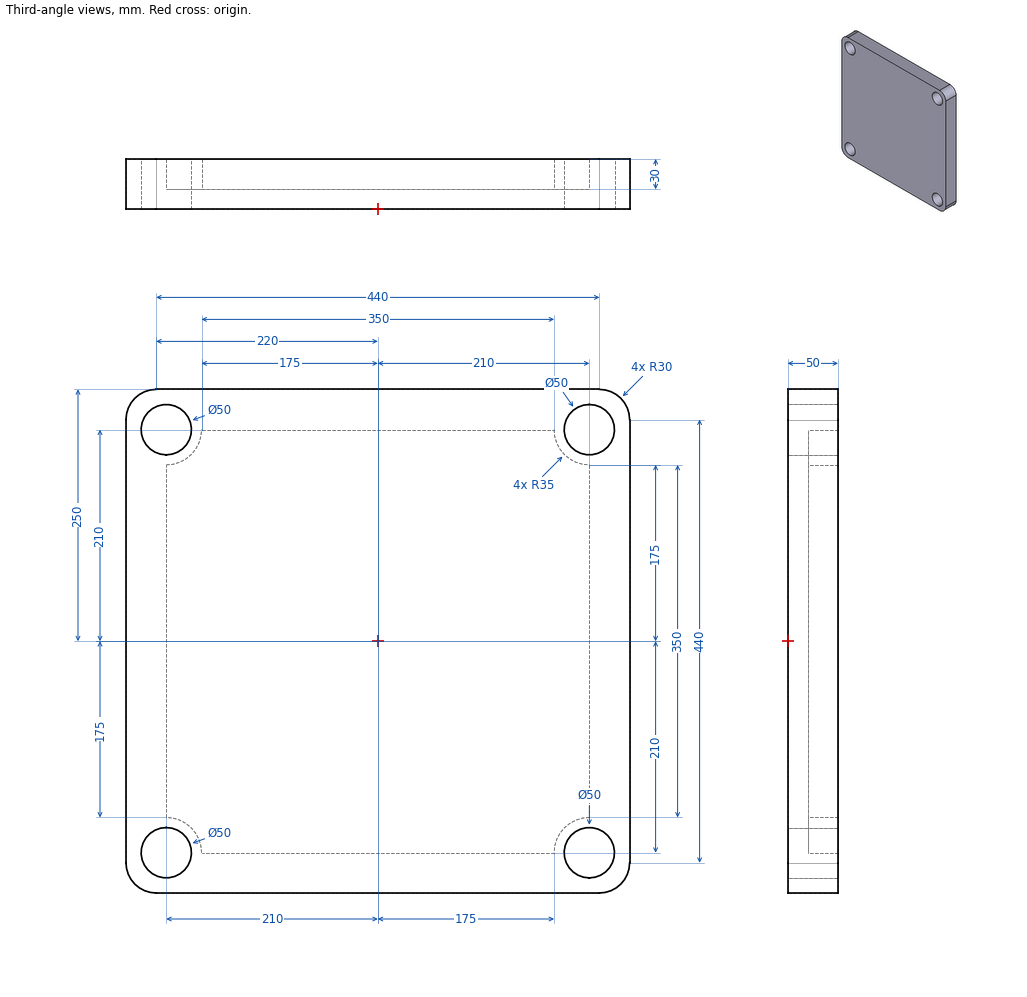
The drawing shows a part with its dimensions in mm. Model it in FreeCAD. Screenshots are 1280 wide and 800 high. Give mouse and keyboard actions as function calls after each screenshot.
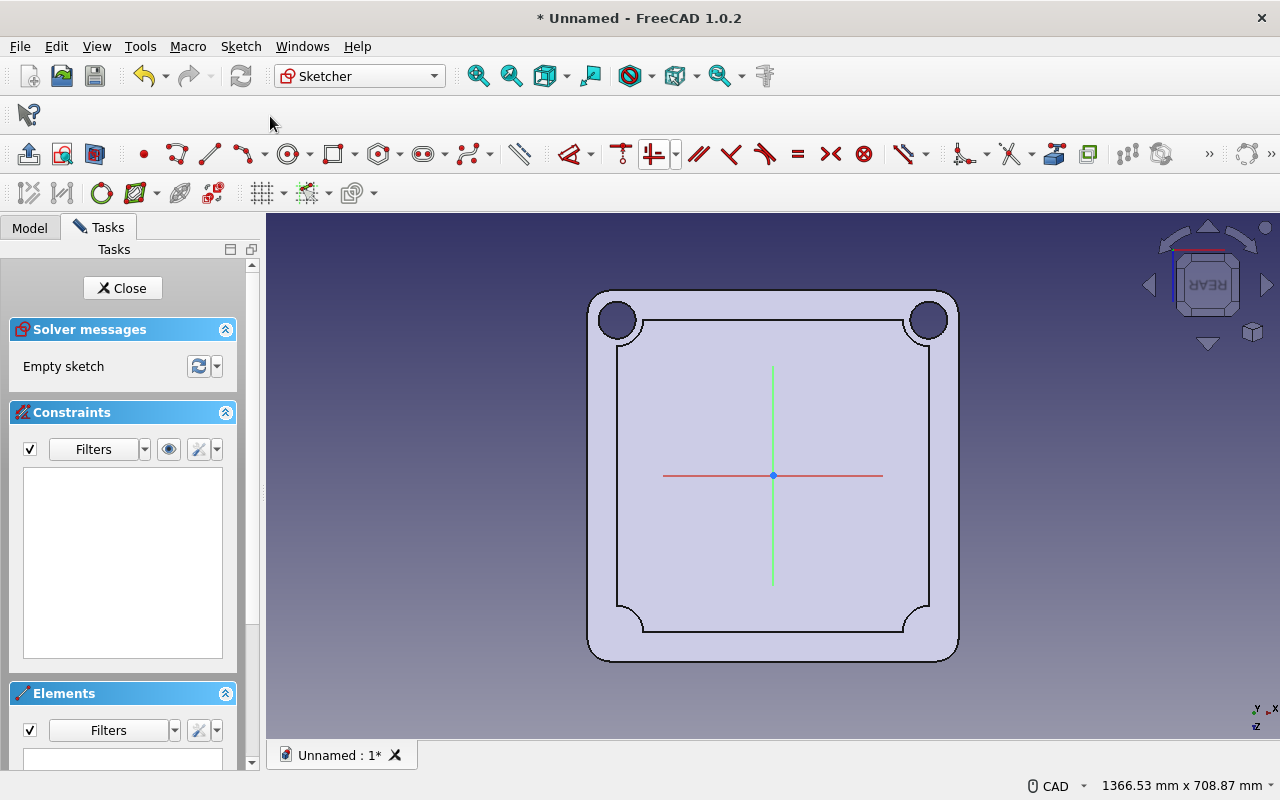
scroll(957, 651, up, 11)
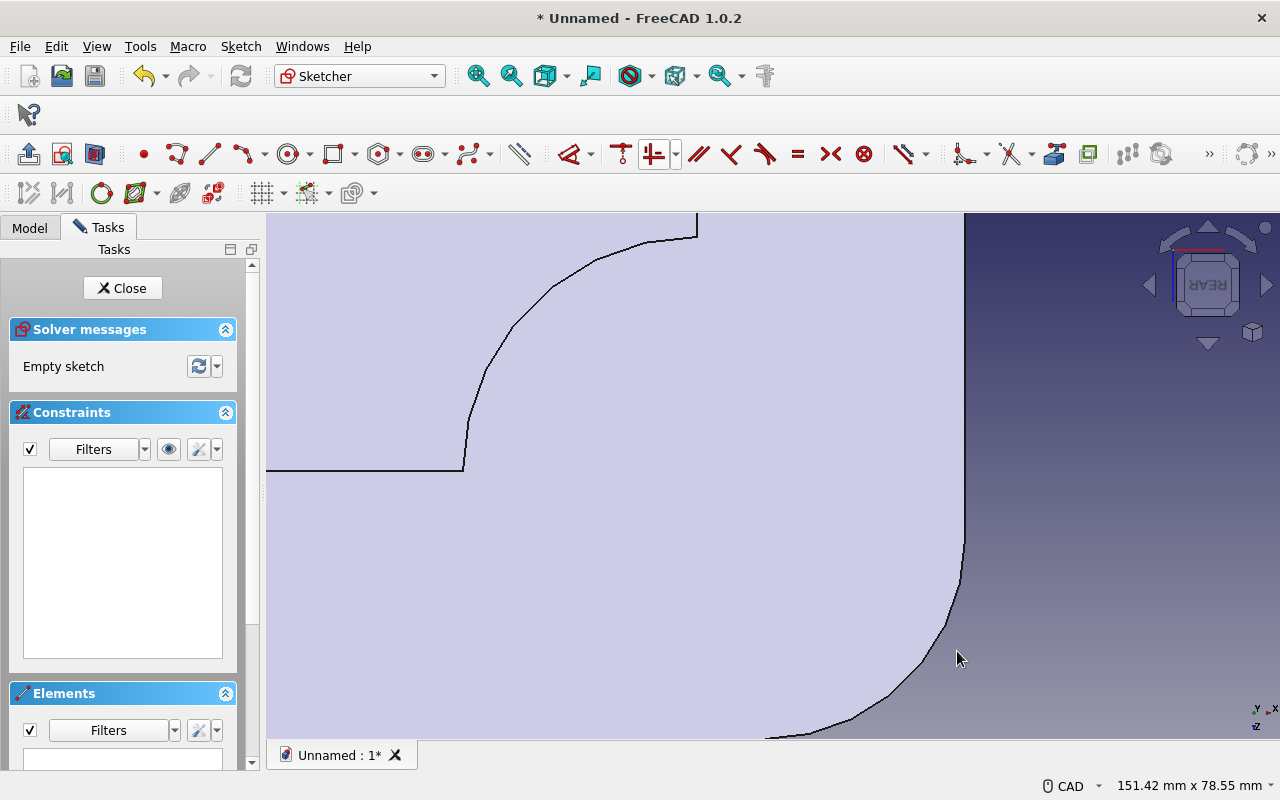
click(288, 154)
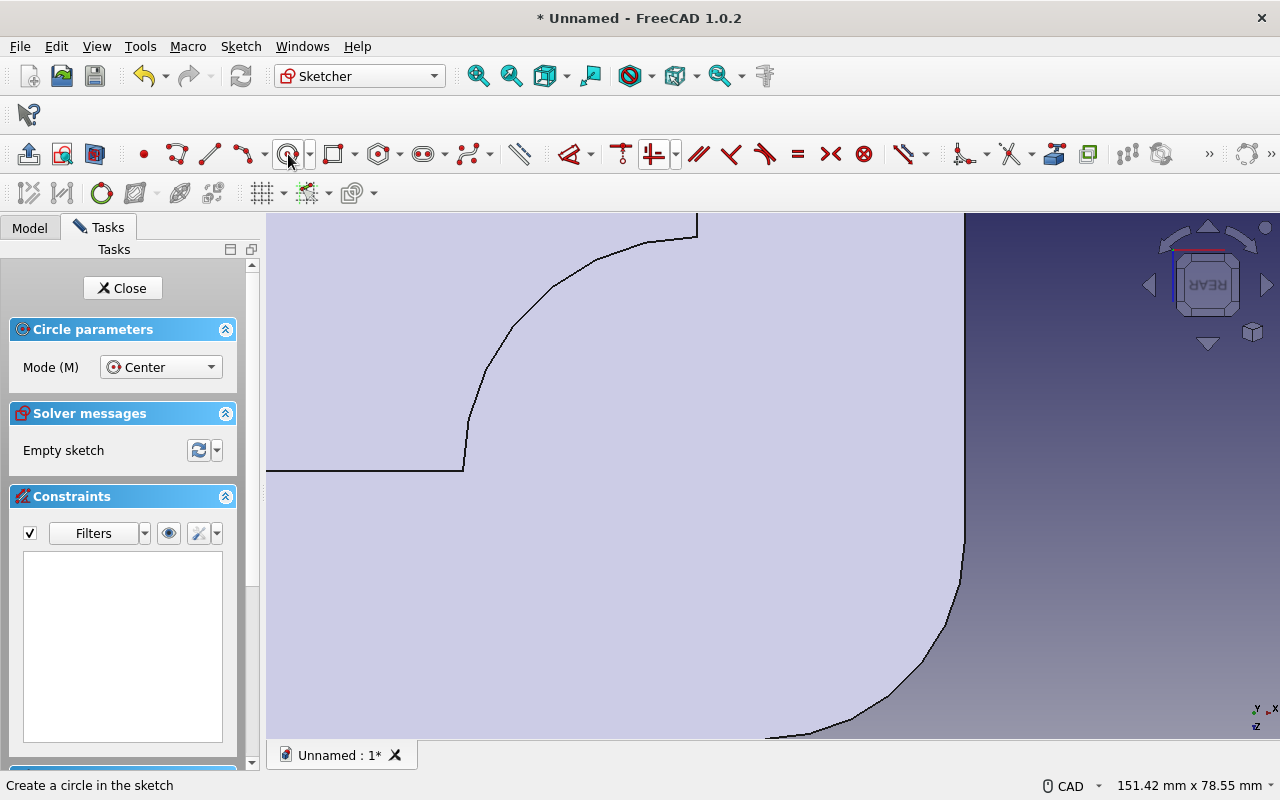
click(697, 471)
move(816, 353)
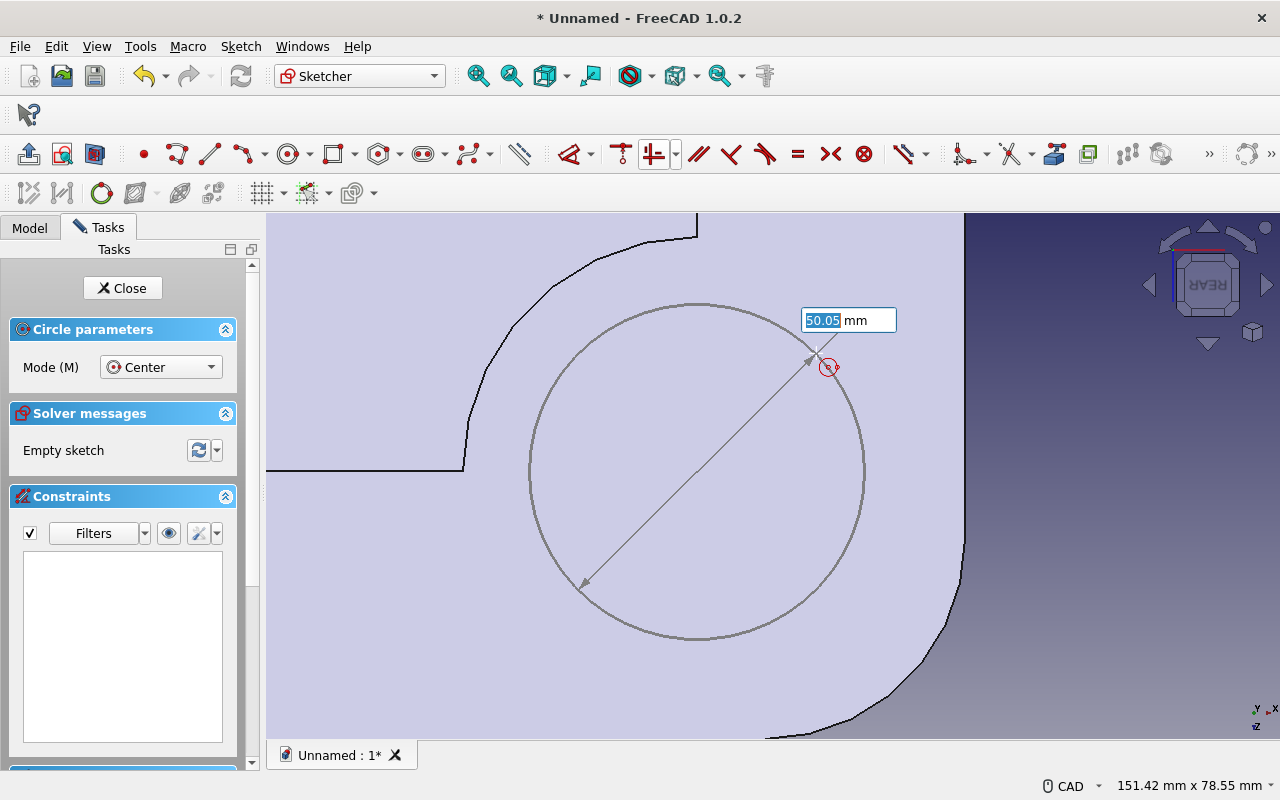
text(50)
key(Return)
key(Escape)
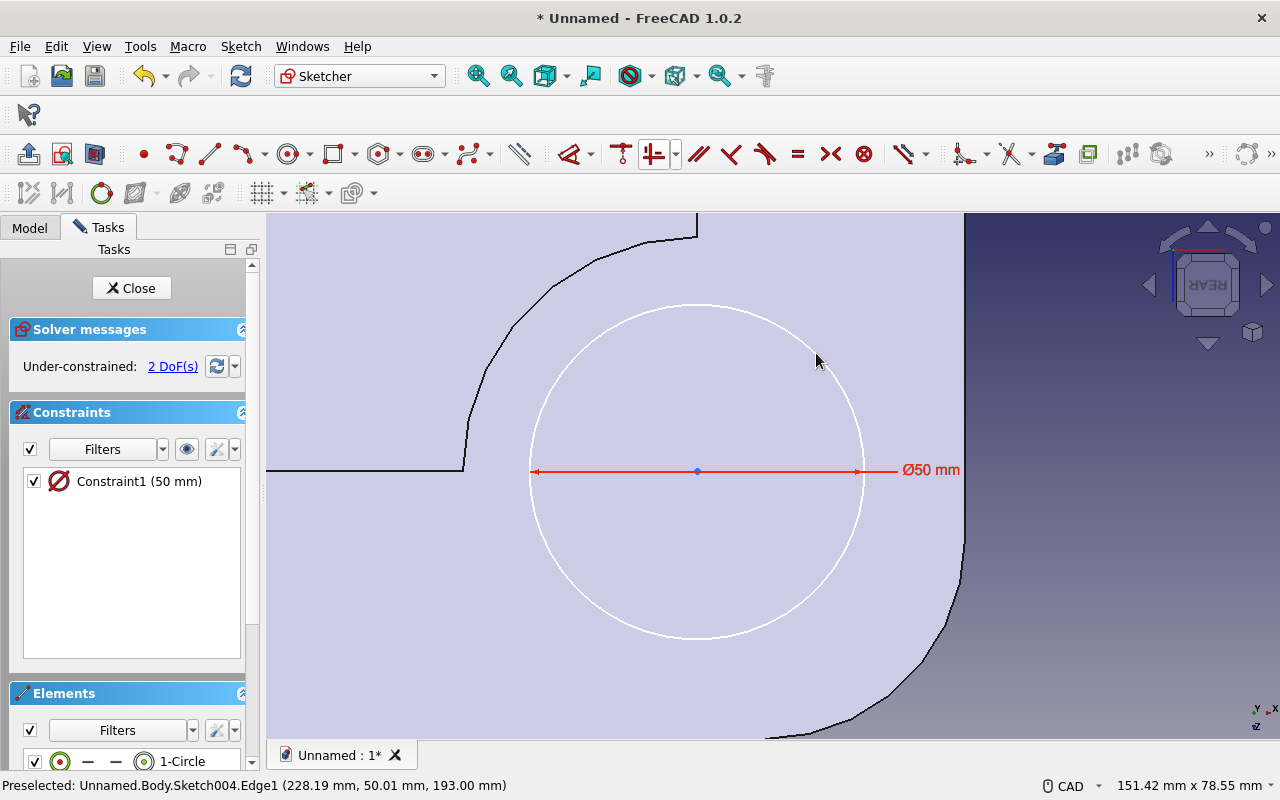
click(568, 154)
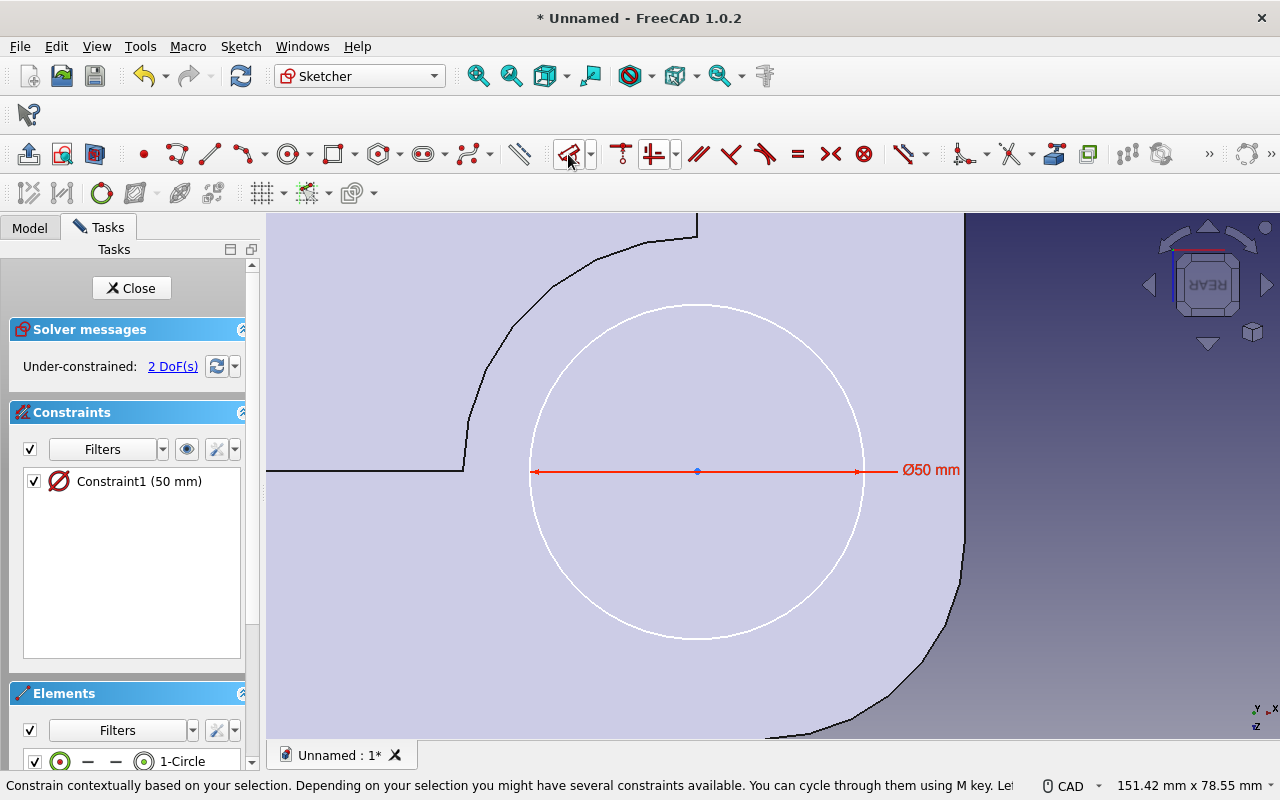
click(697, 472)
click(495, 506)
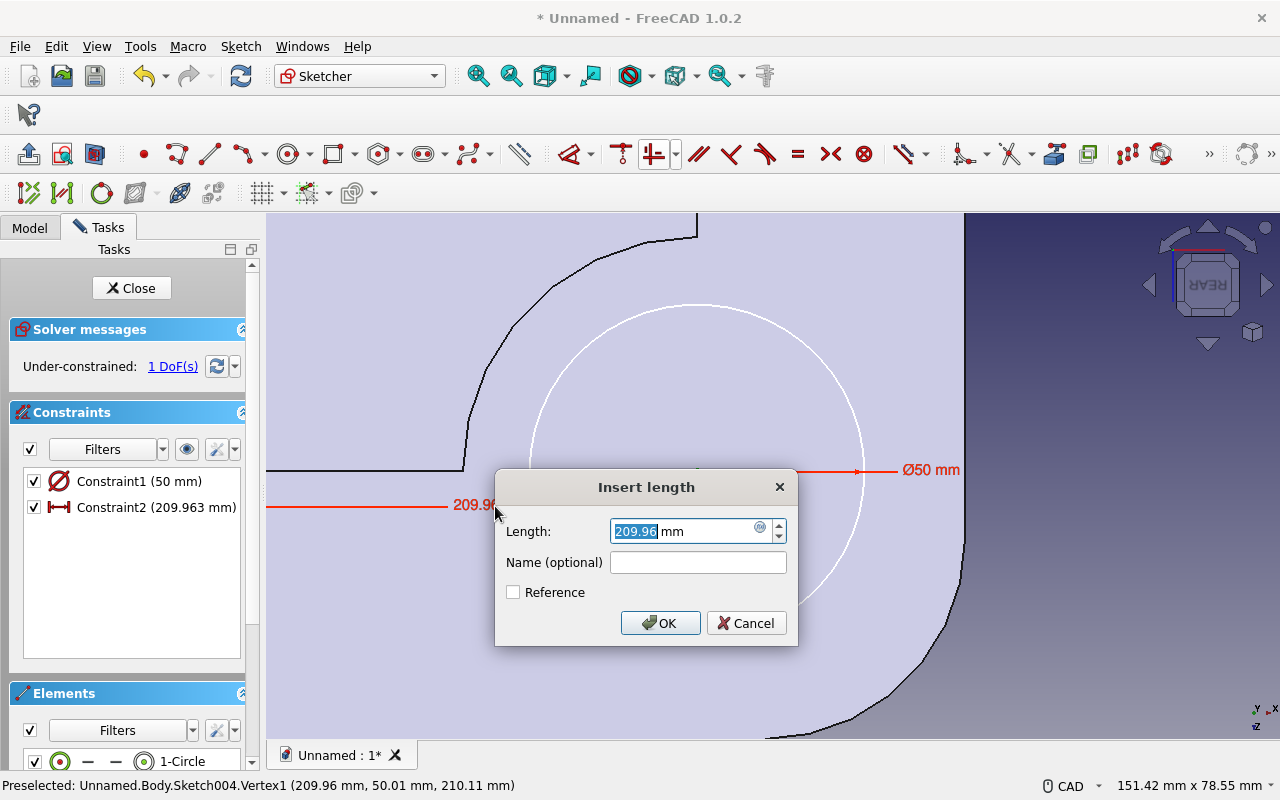
text(210)
key(Return)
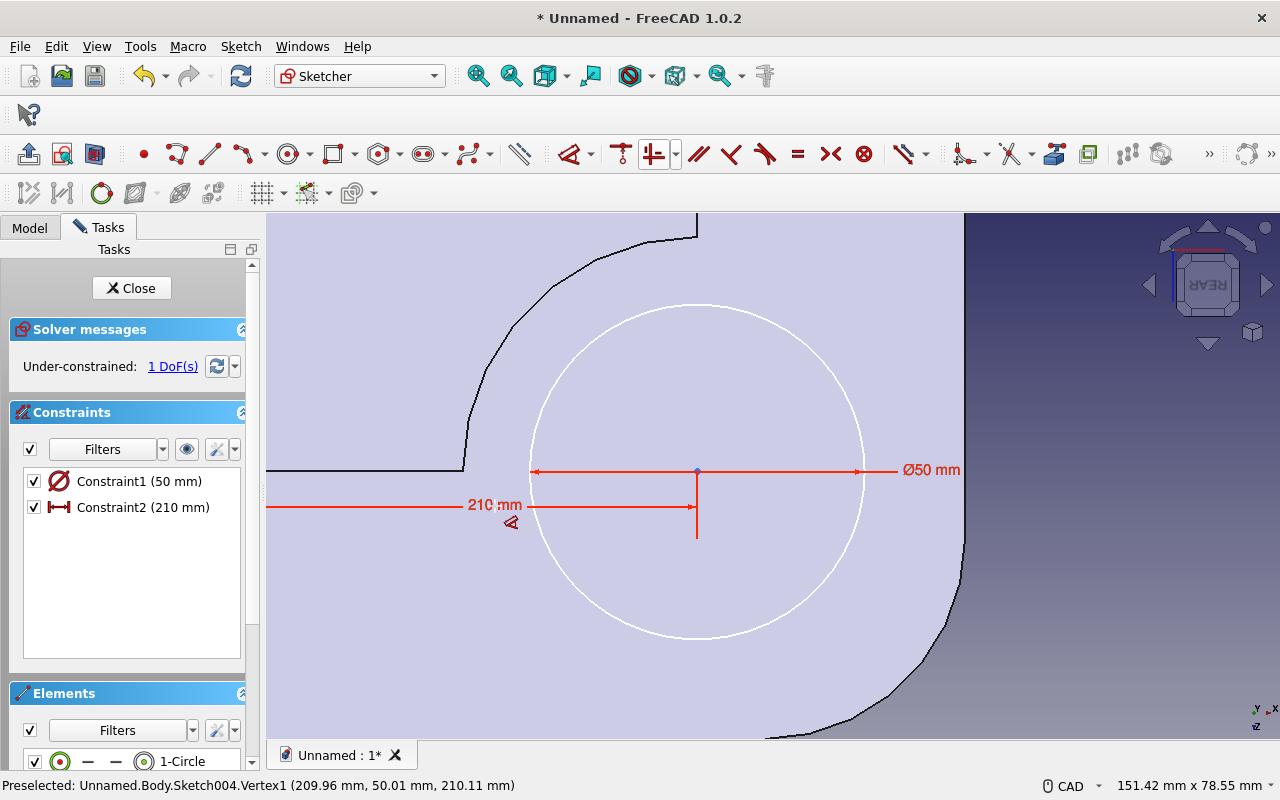
click(697, 472)
click(731, 356)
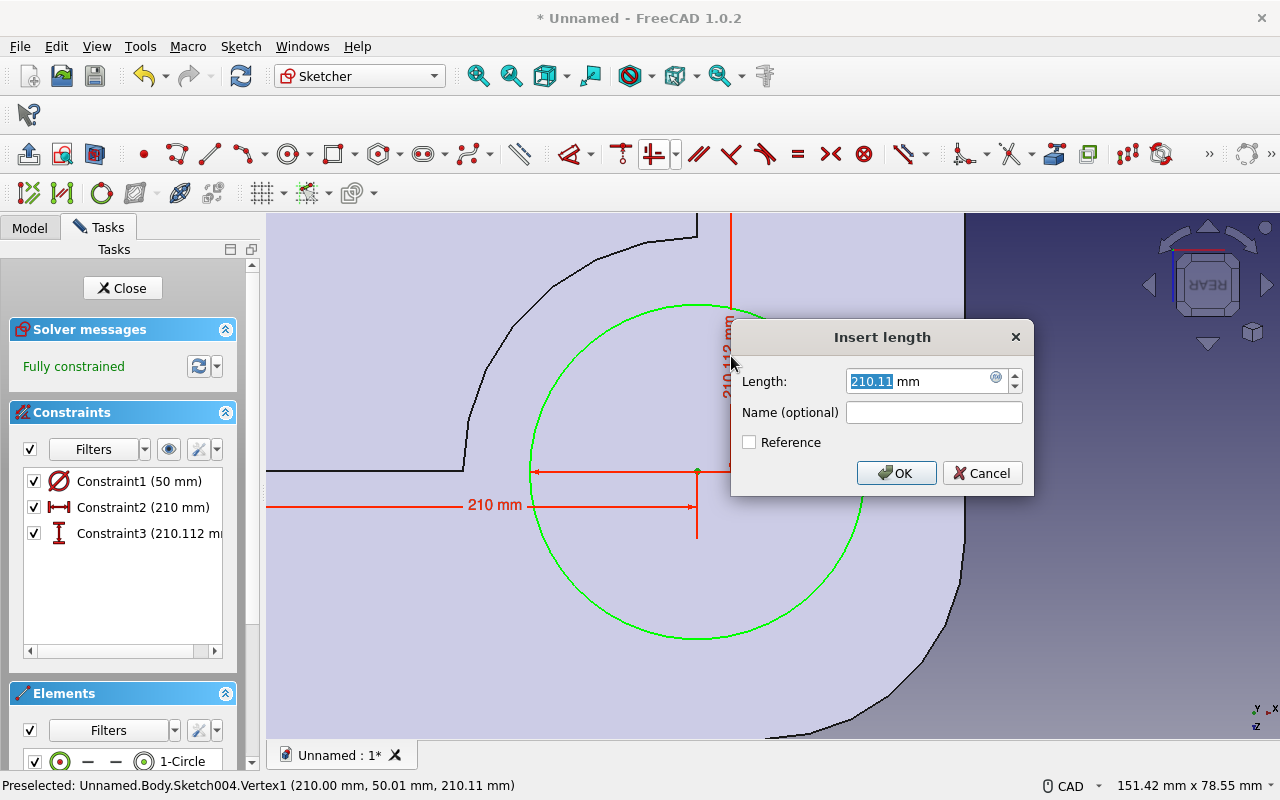
text(210)
key(Return)
key(Escape)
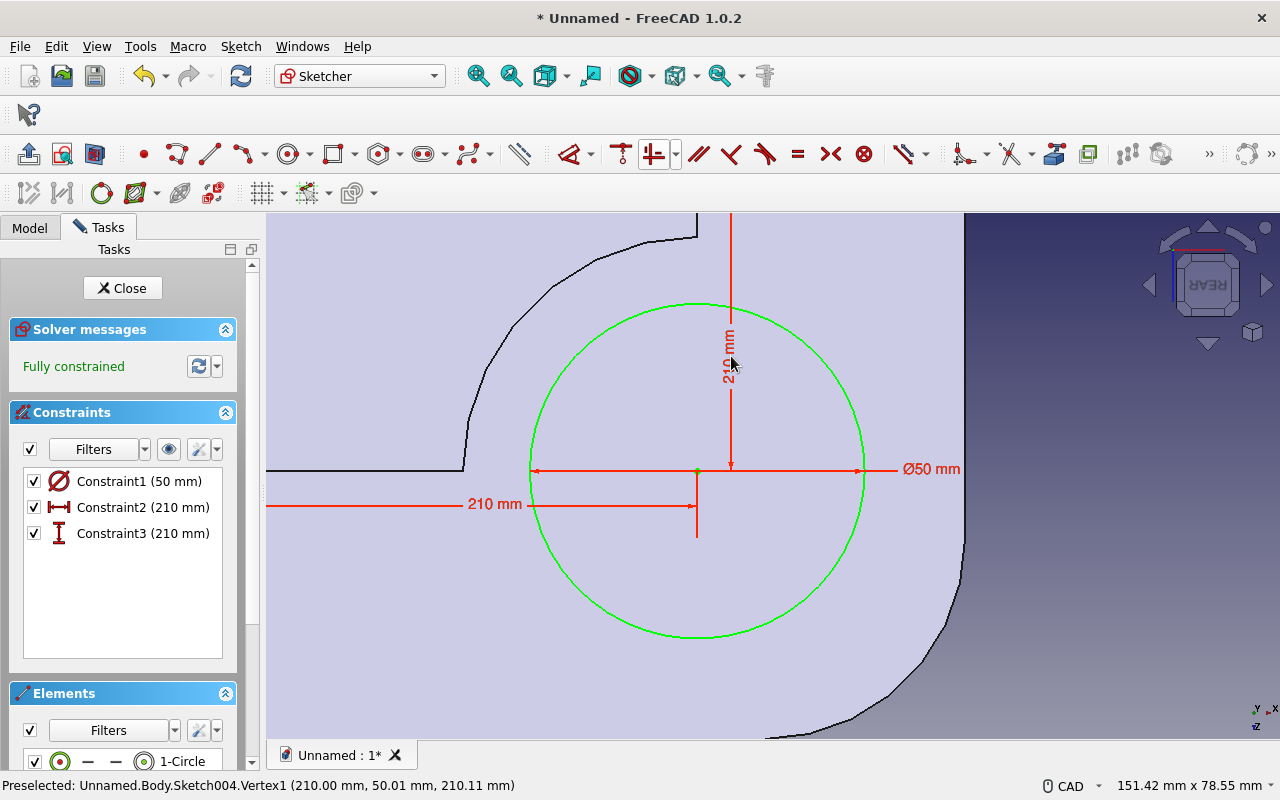
click(123, 288)